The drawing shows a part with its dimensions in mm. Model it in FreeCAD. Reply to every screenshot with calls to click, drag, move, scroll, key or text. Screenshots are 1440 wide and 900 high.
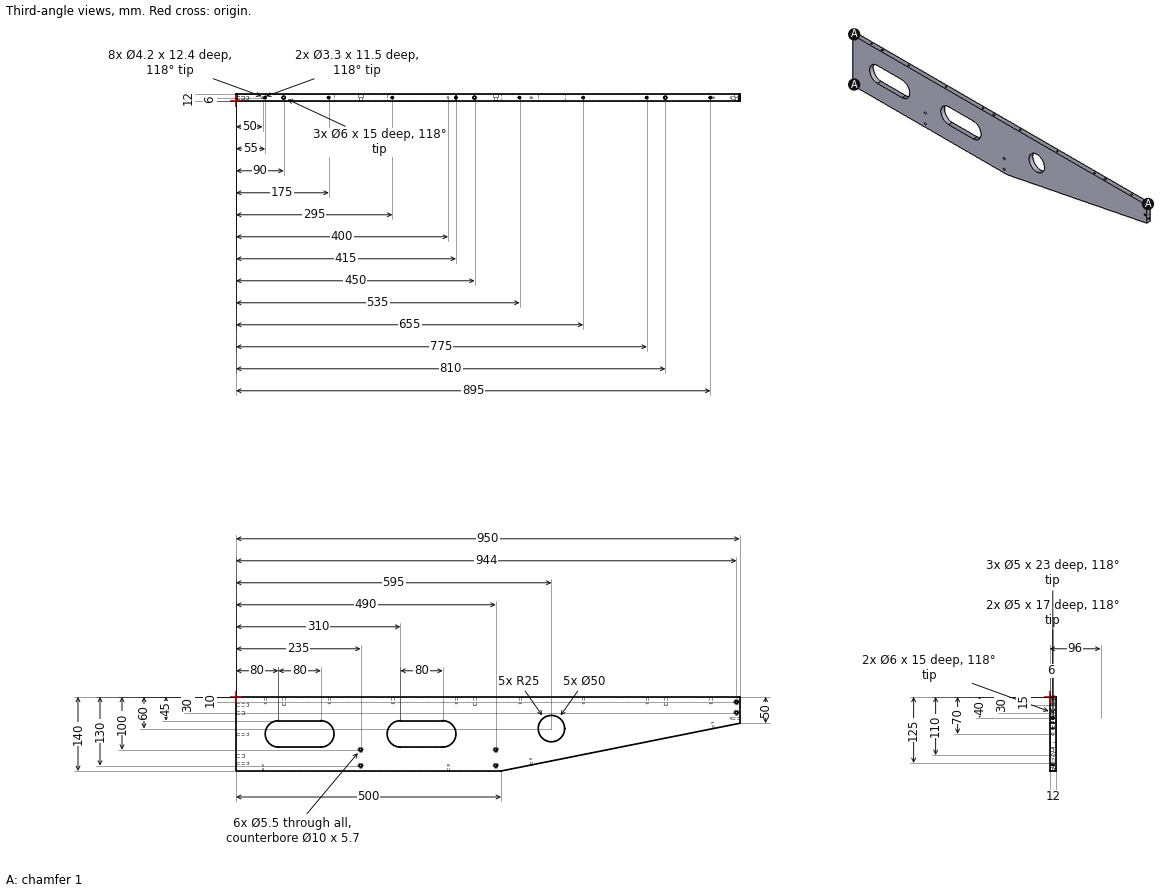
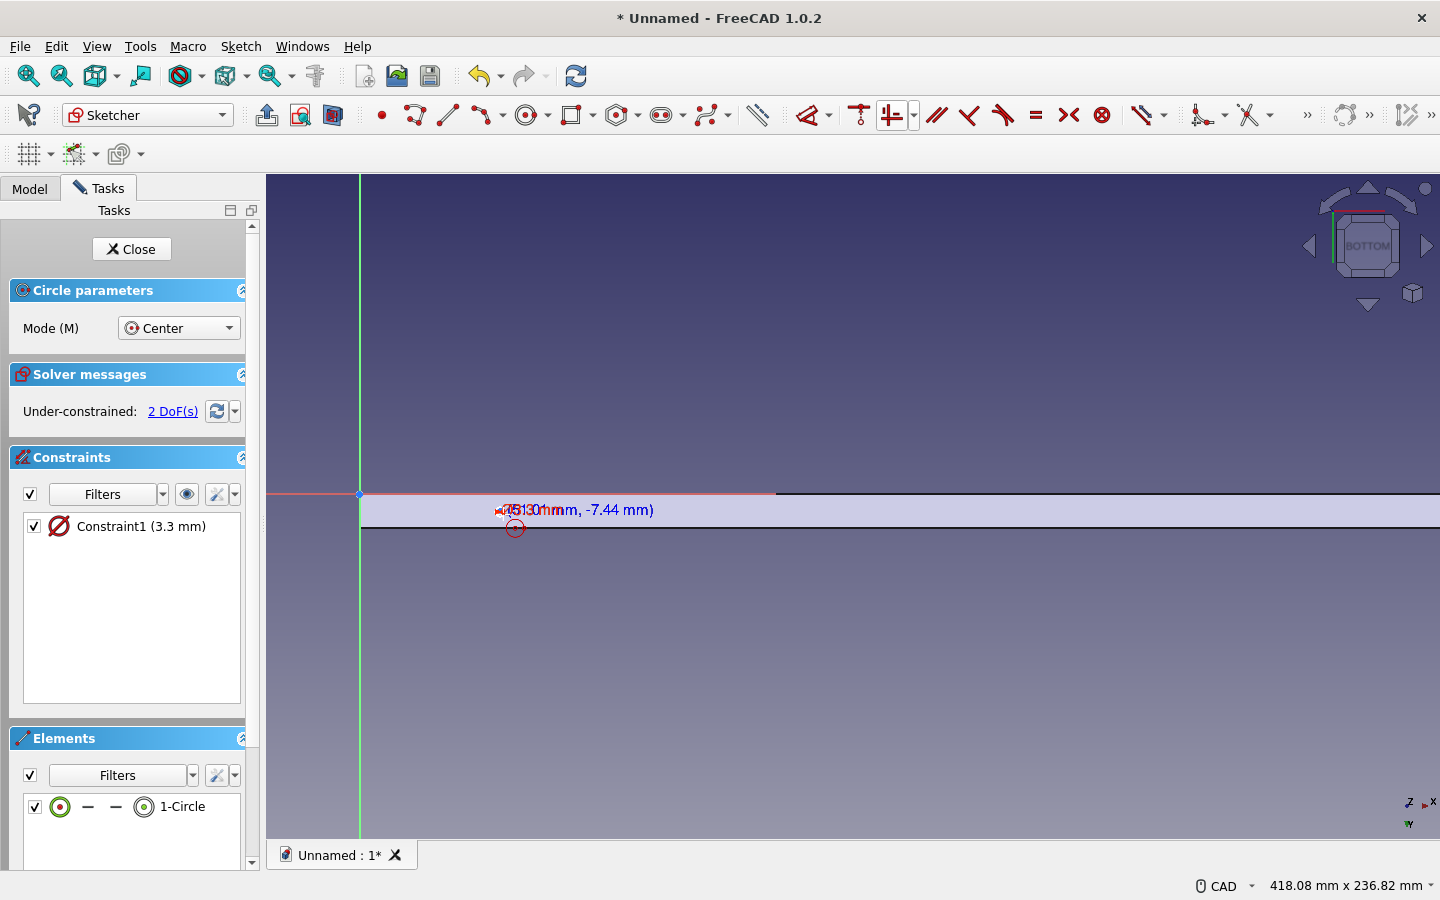
scroll(501, 510, down, 2)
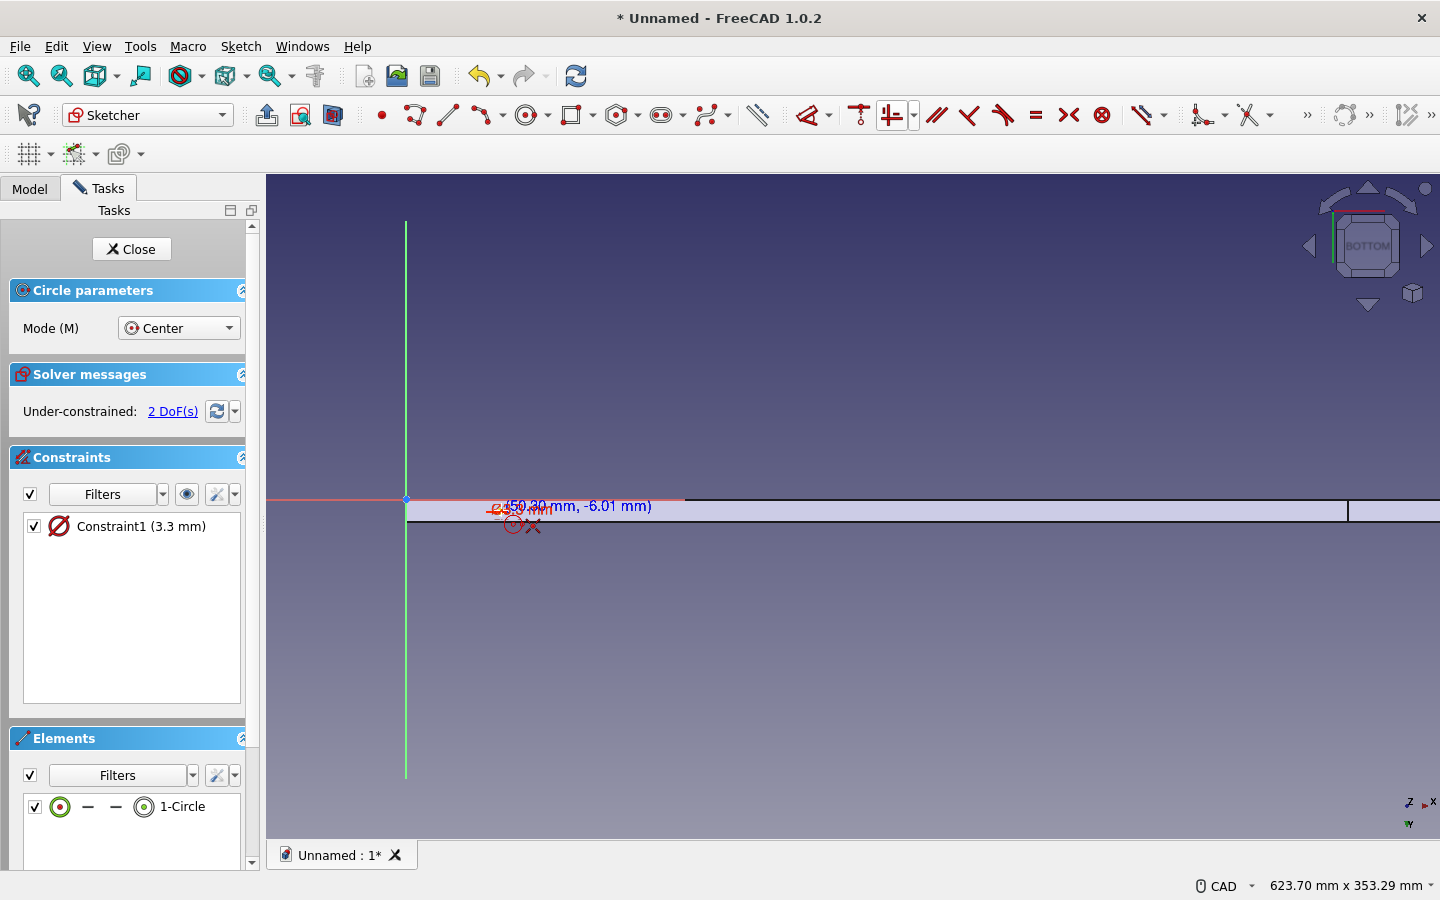
scroll(1159, 511, up, 10)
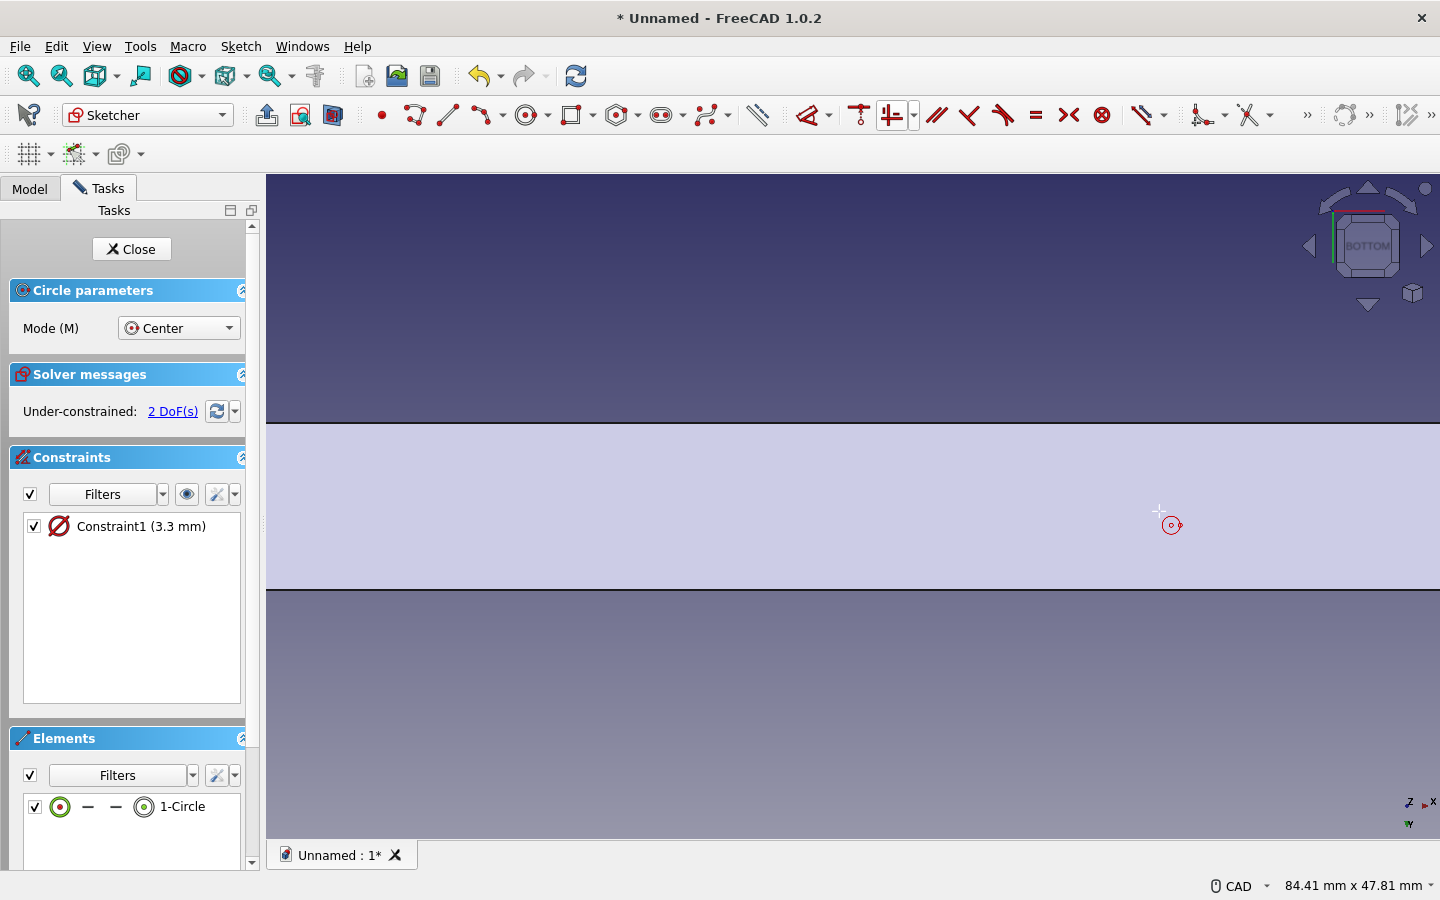
scroll(1160, 511, down, 10)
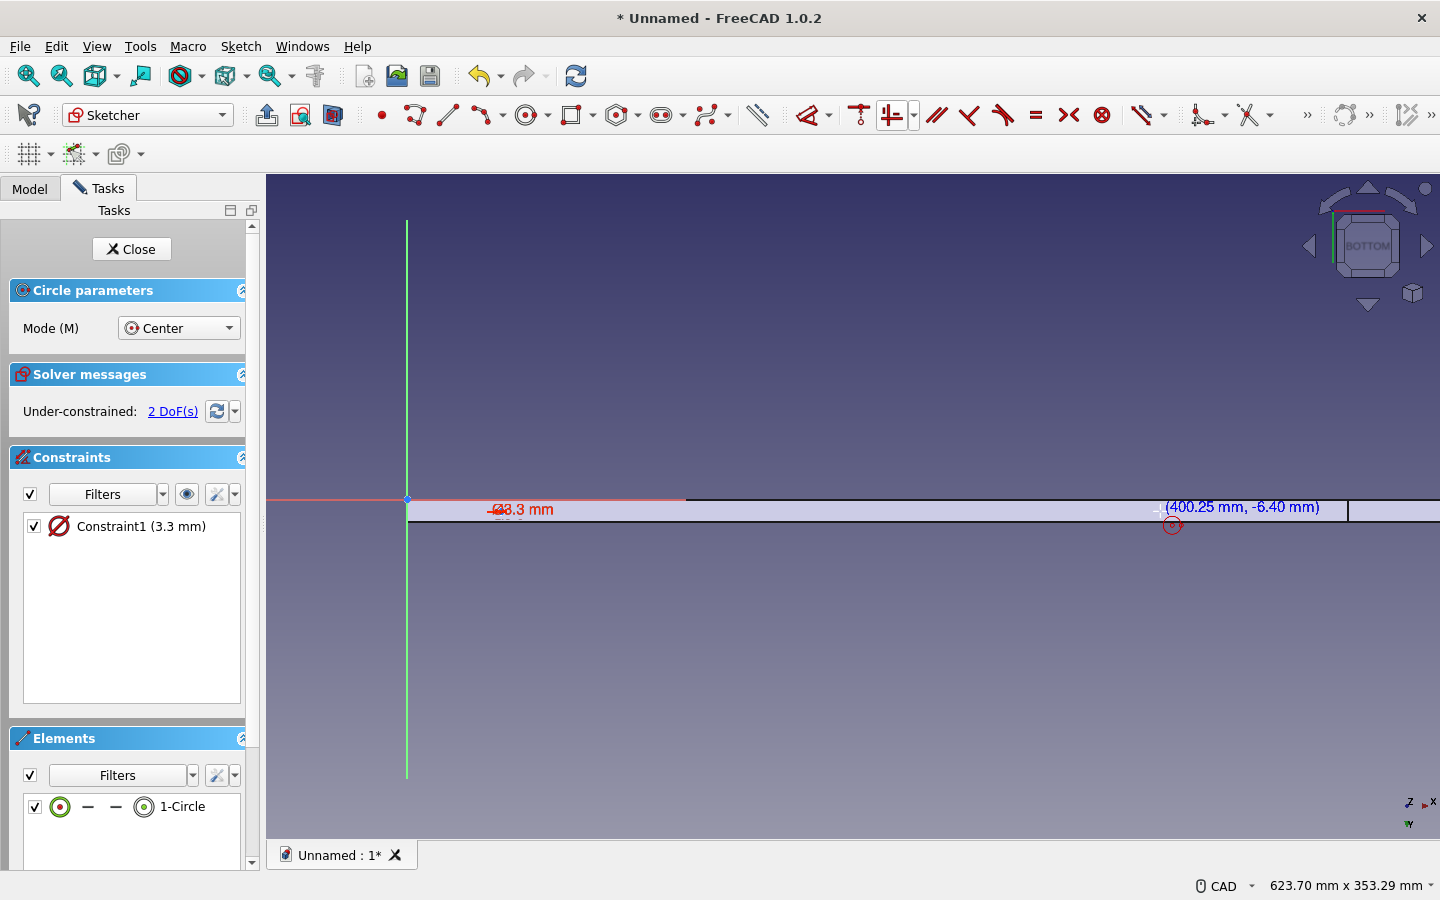
scroll(1160, 511, up, 2)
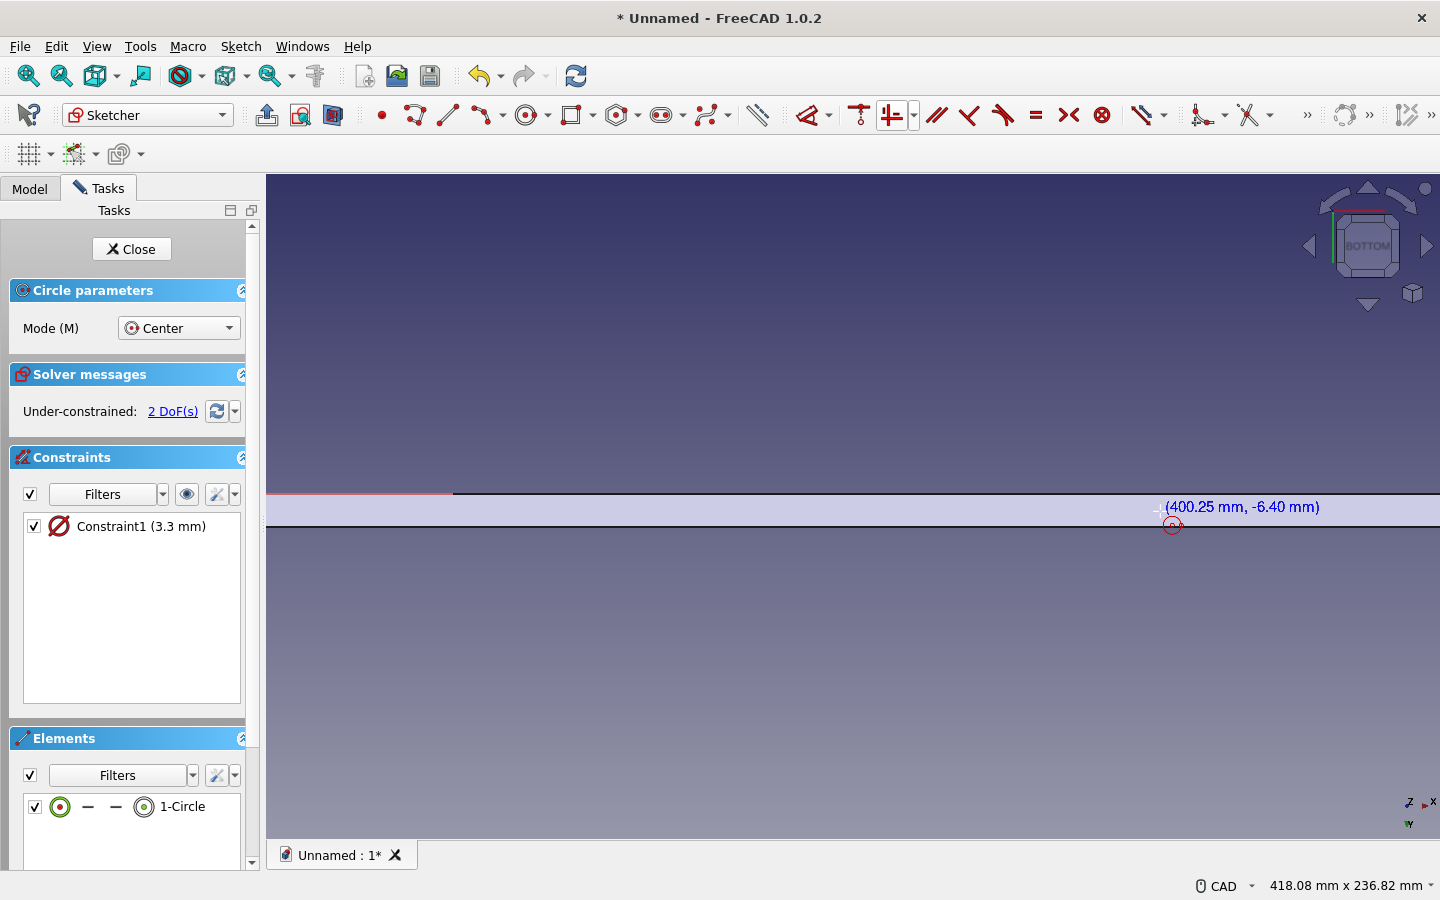
click(1160, 510)
move(1163, 514)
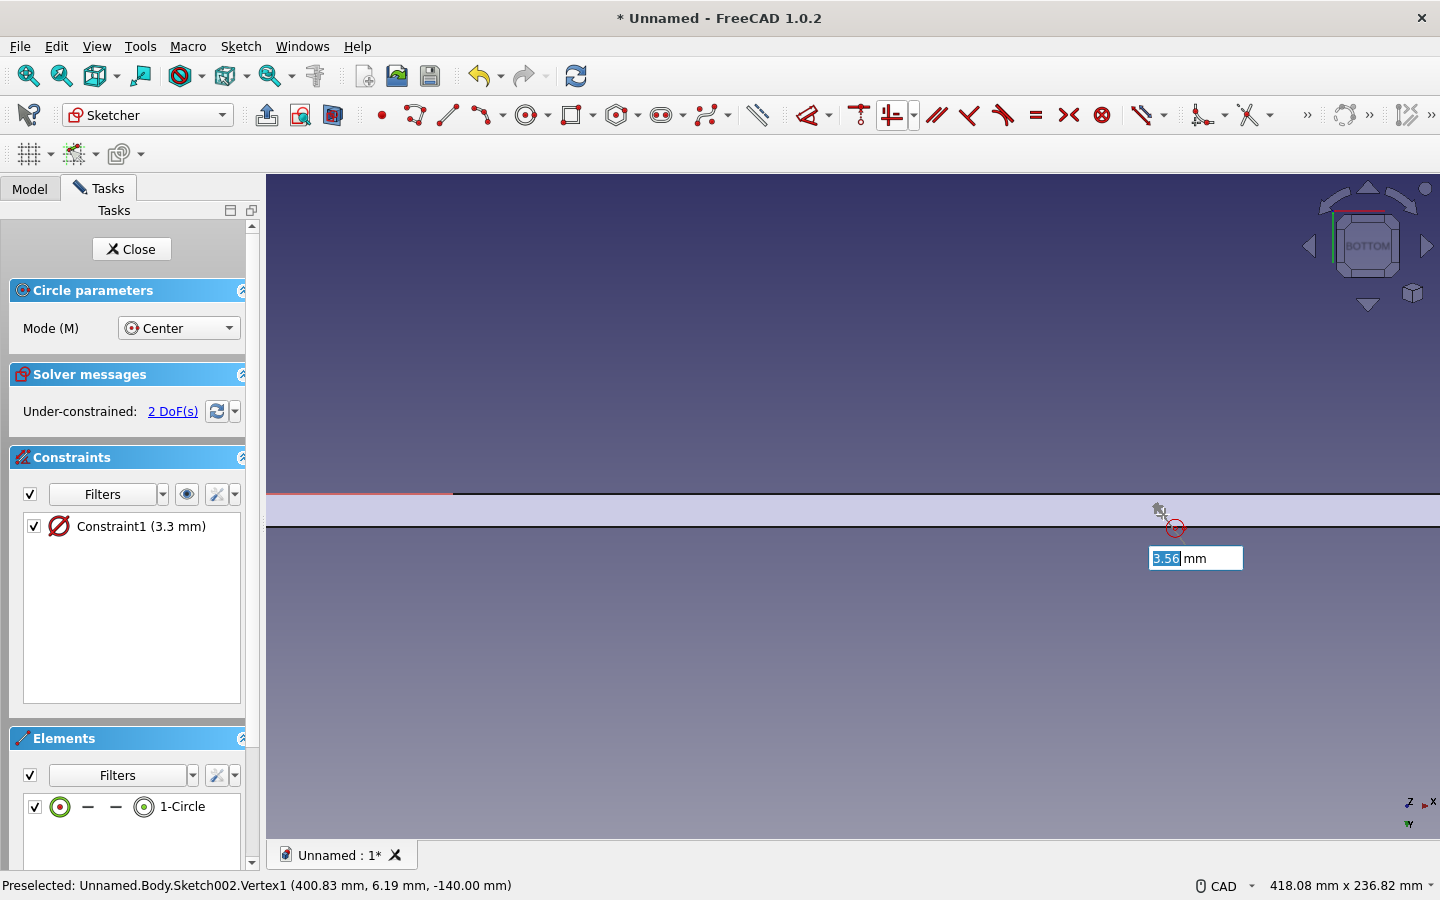
text(3.3)
key(Return)
key(Escape)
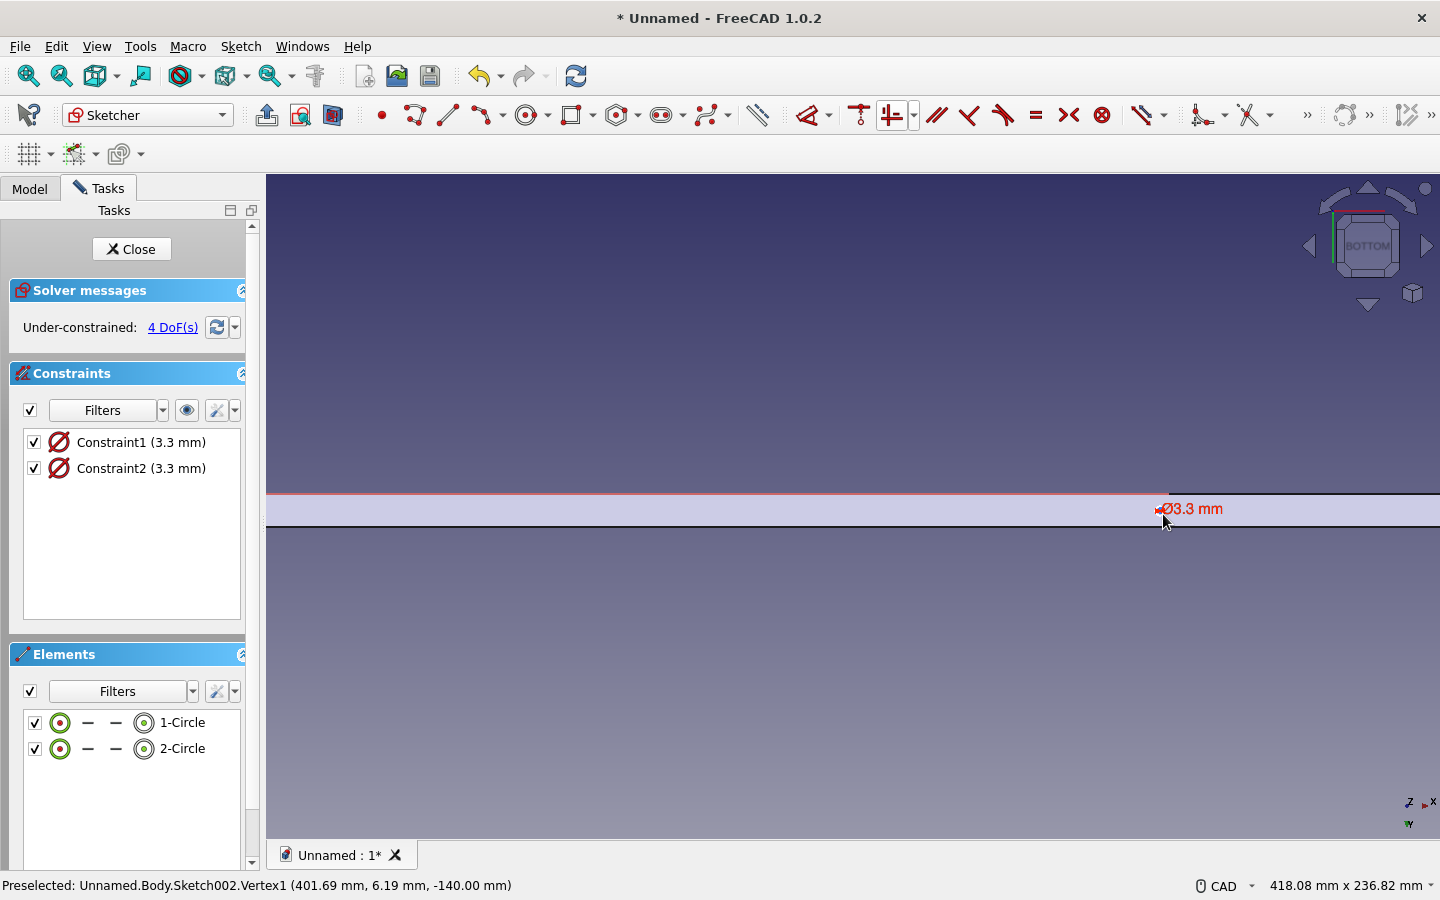
click(806, 116)